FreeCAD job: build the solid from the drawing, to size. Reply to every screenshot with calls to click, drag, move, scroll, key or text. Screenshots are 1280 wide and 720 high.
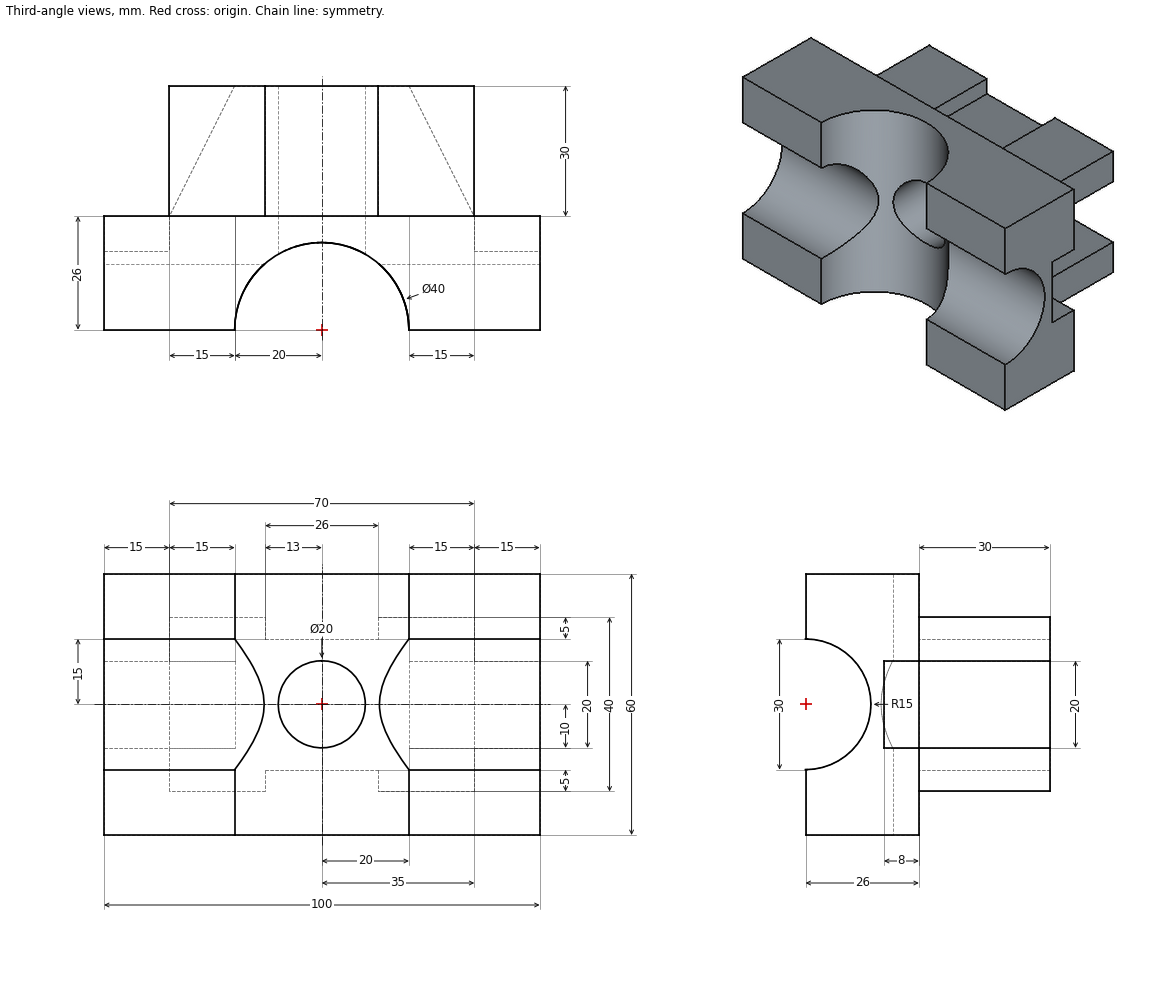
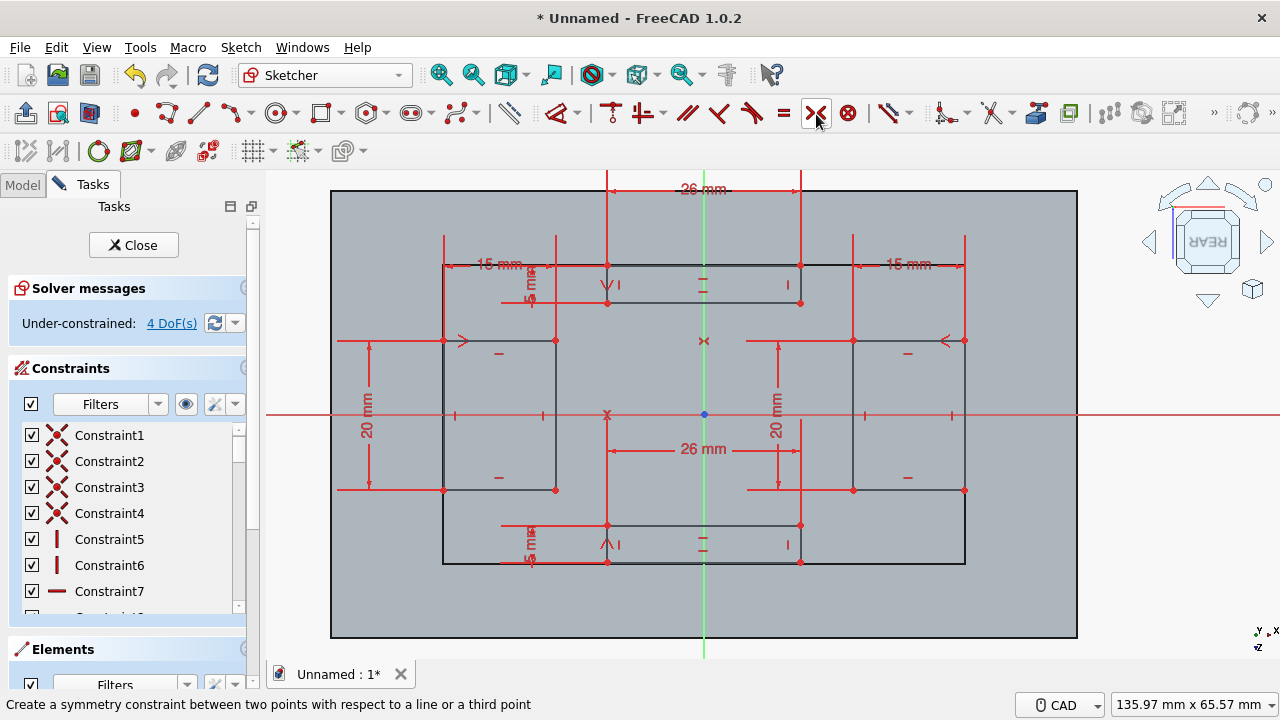
key(d)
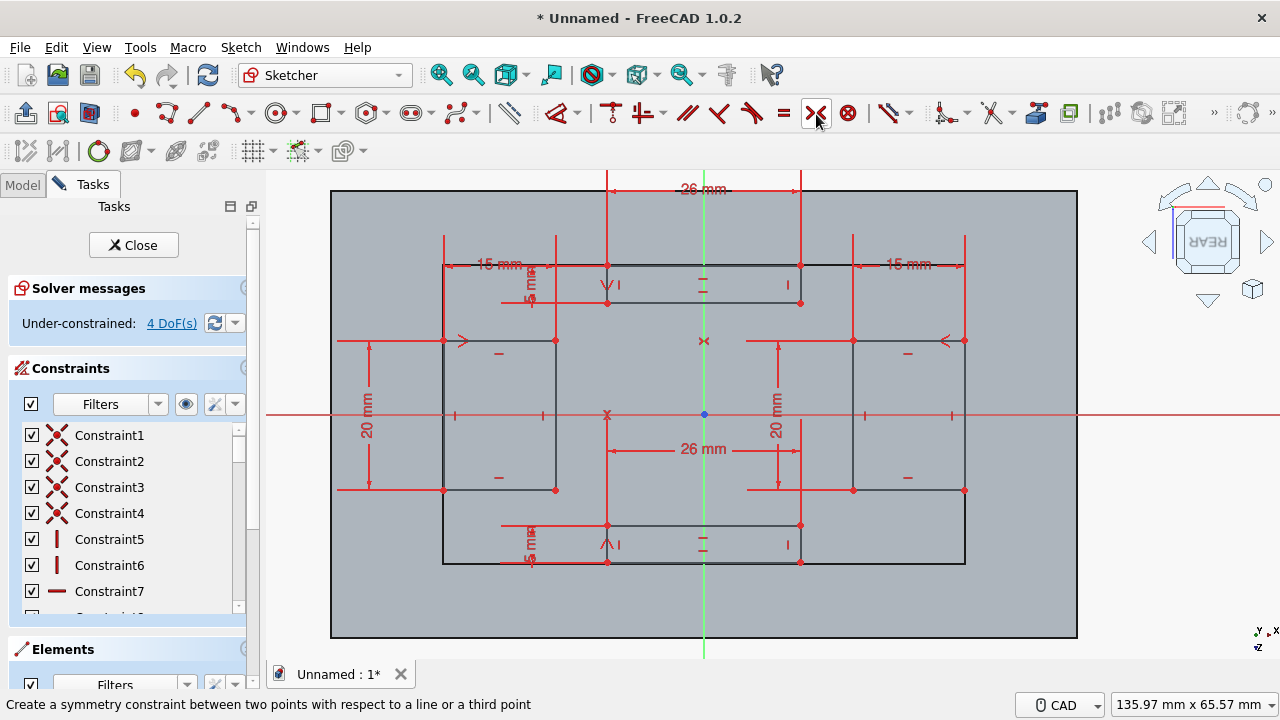
click(853, 341)
click(831, 307)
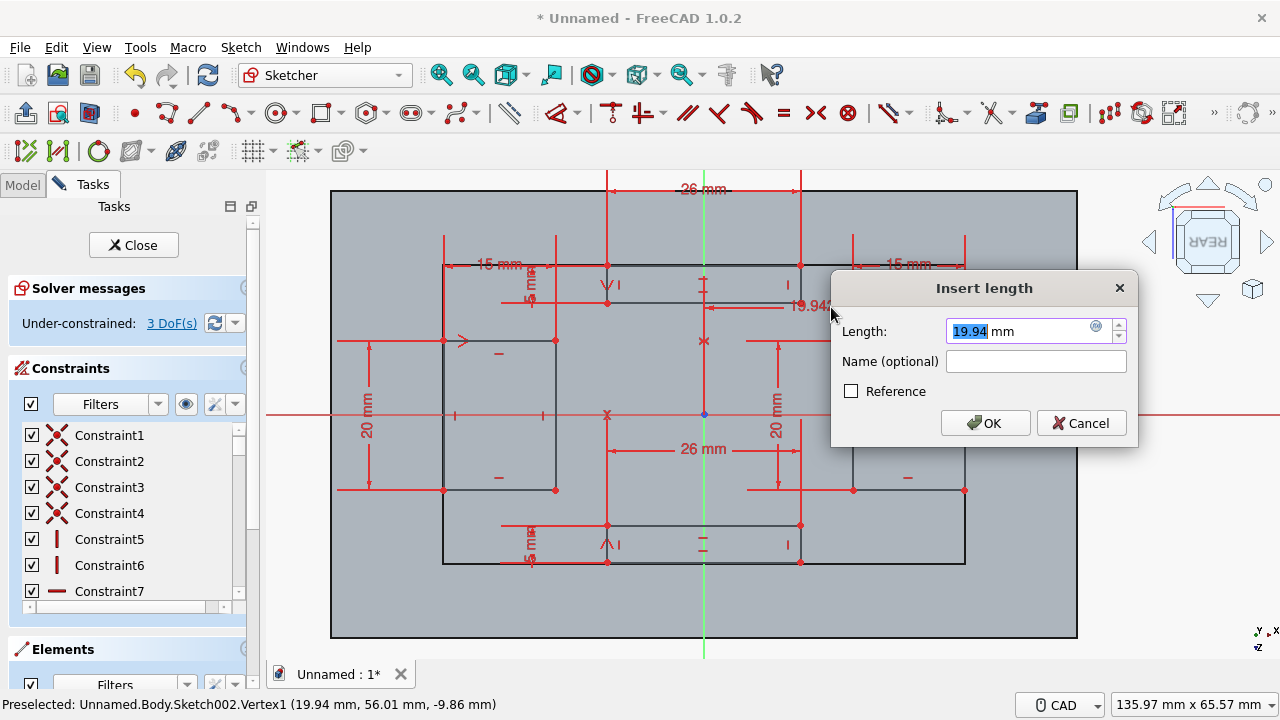
text(20)
key(Return)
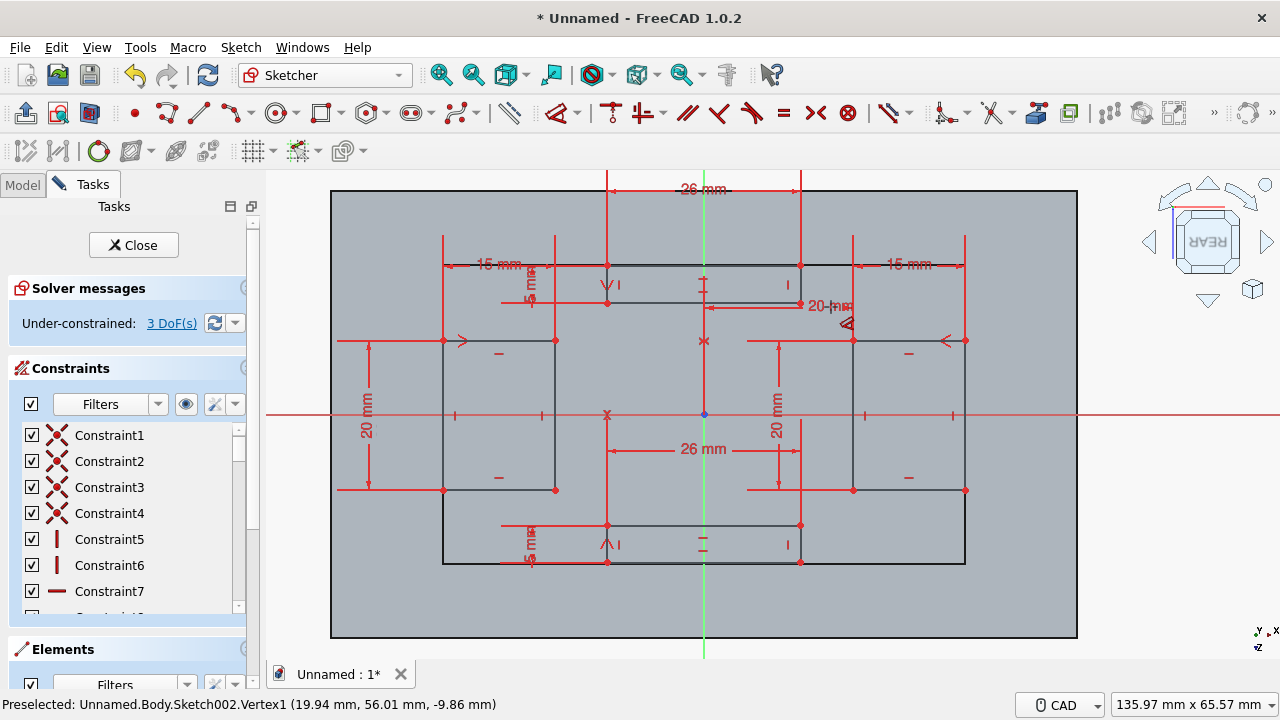
click(853, 341)
click(887, 378)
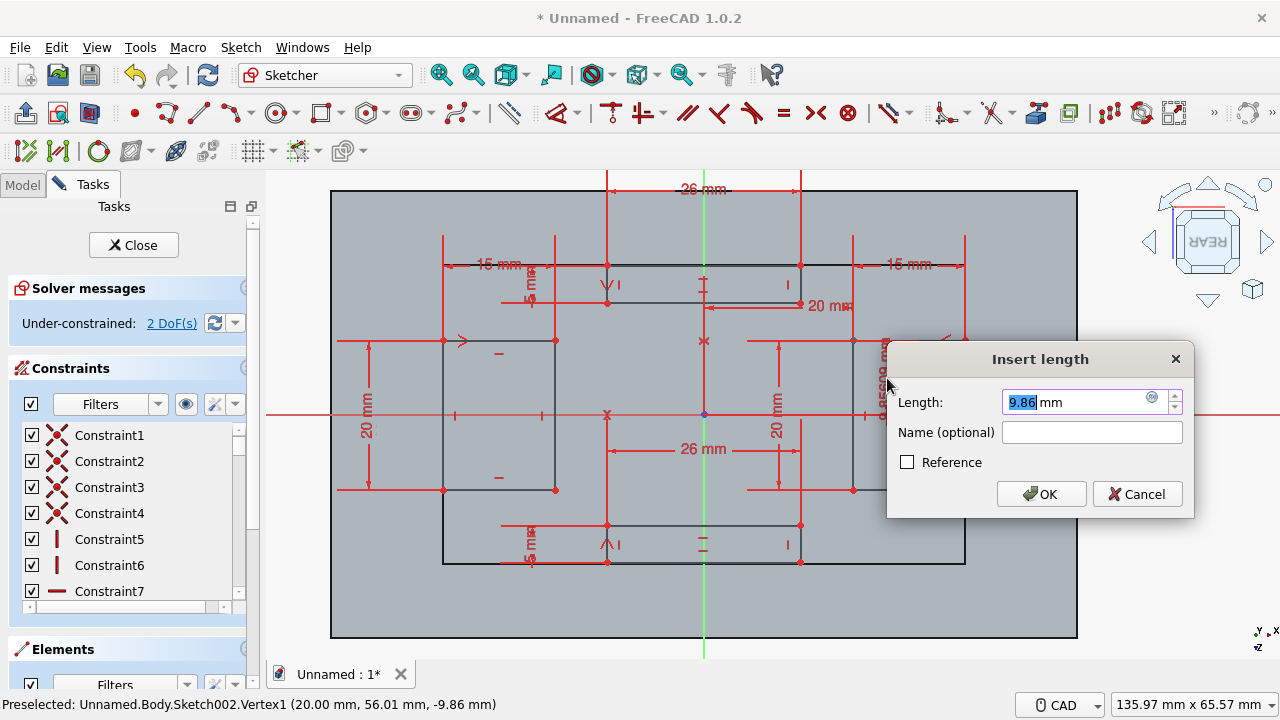
text(10)
key(Return)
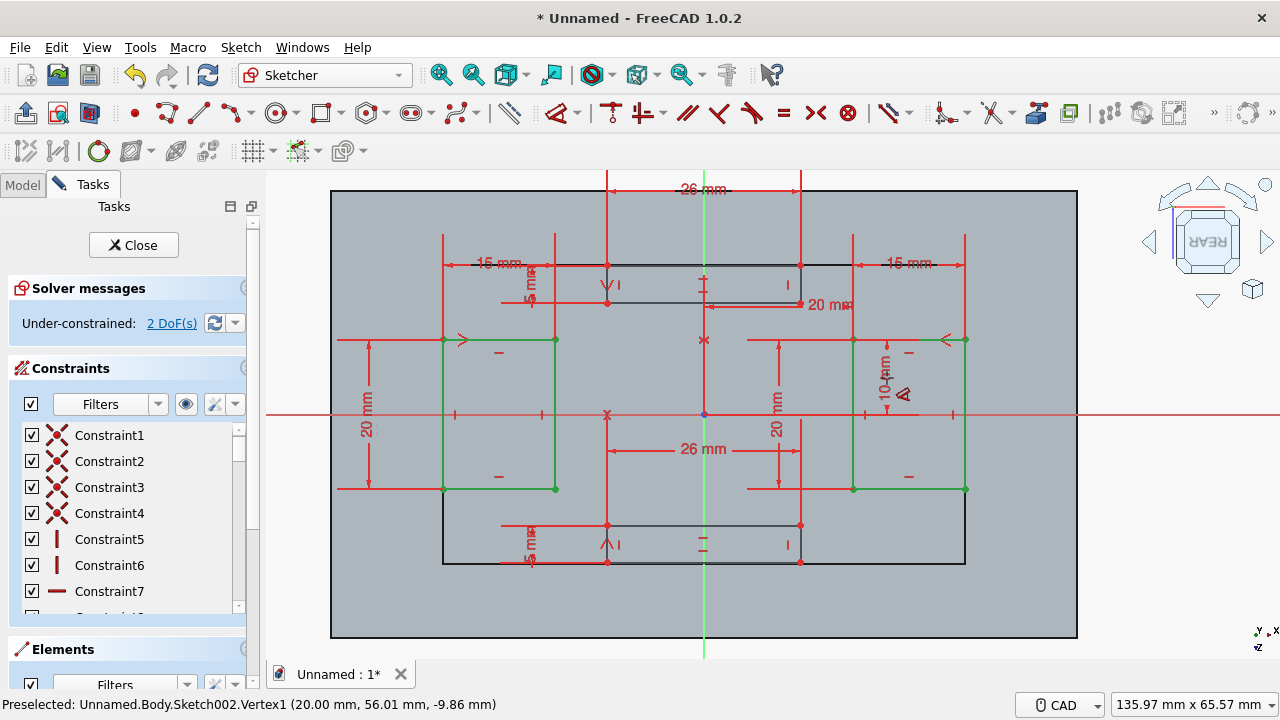
click(607, 526)
click(656, 380)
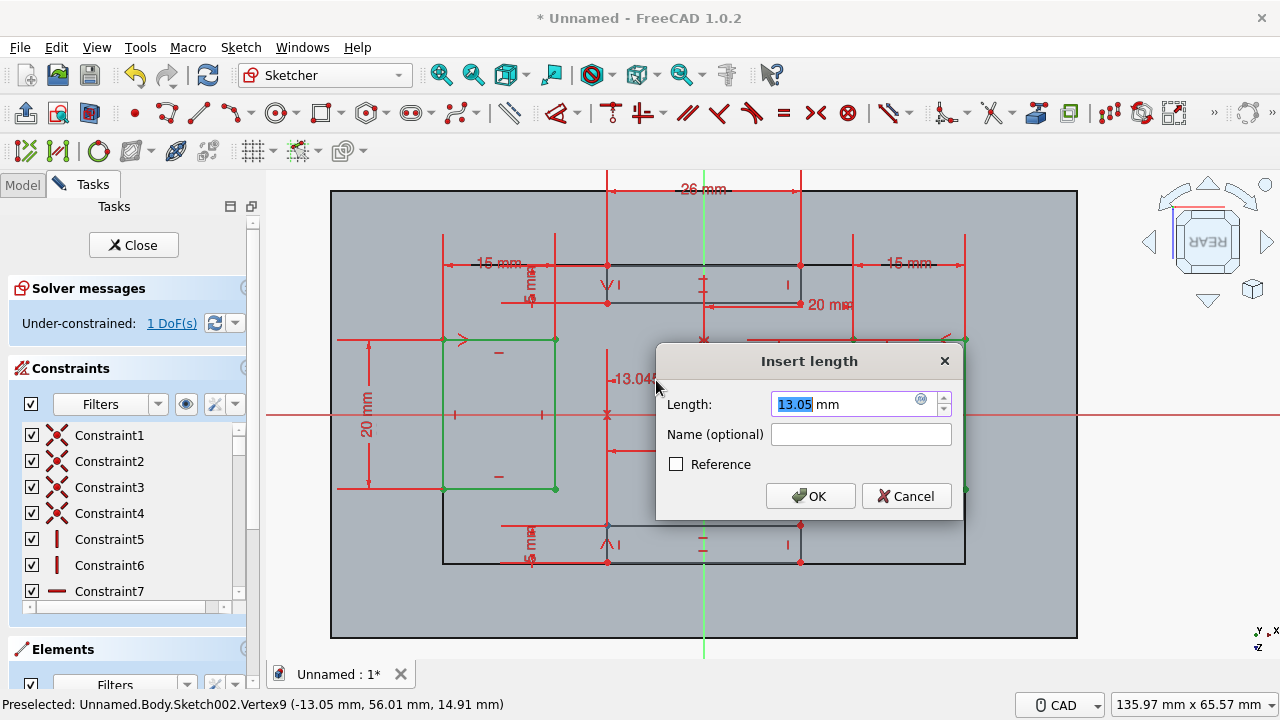
text(13)
key(Return)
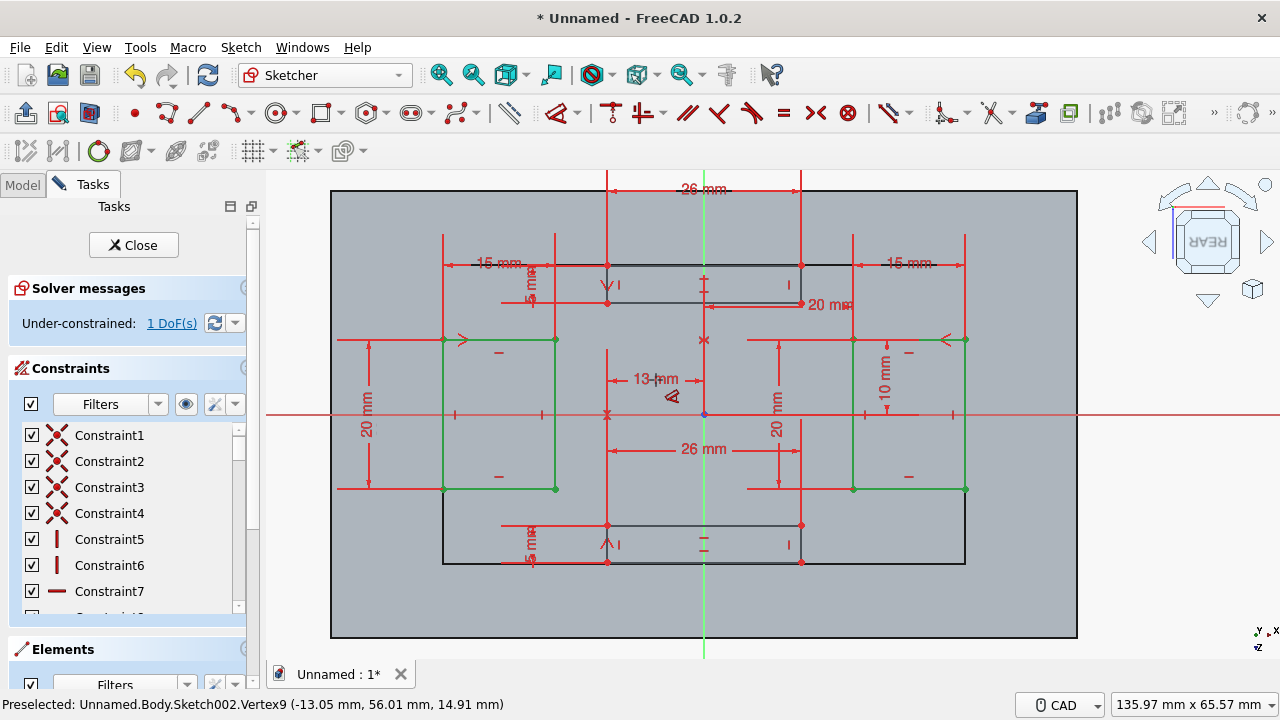
click(607, 526)
click(573, 470)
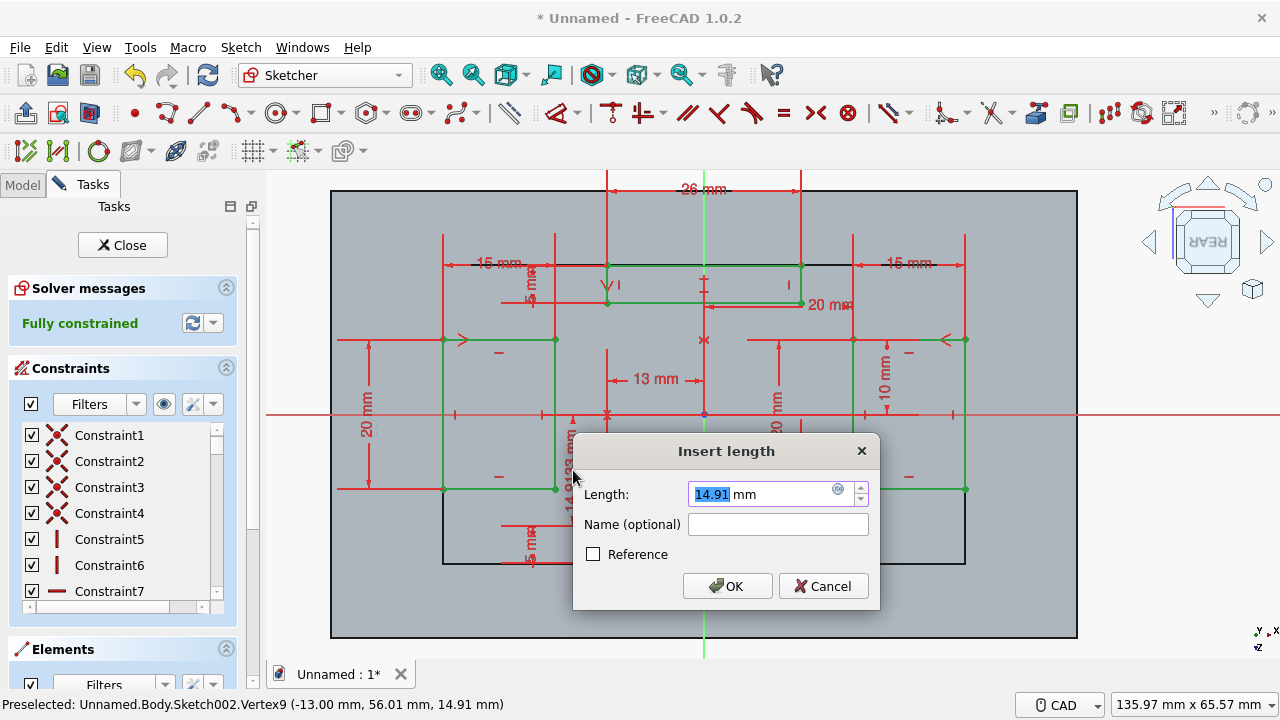
text(15)
key(Return)
key(Escape)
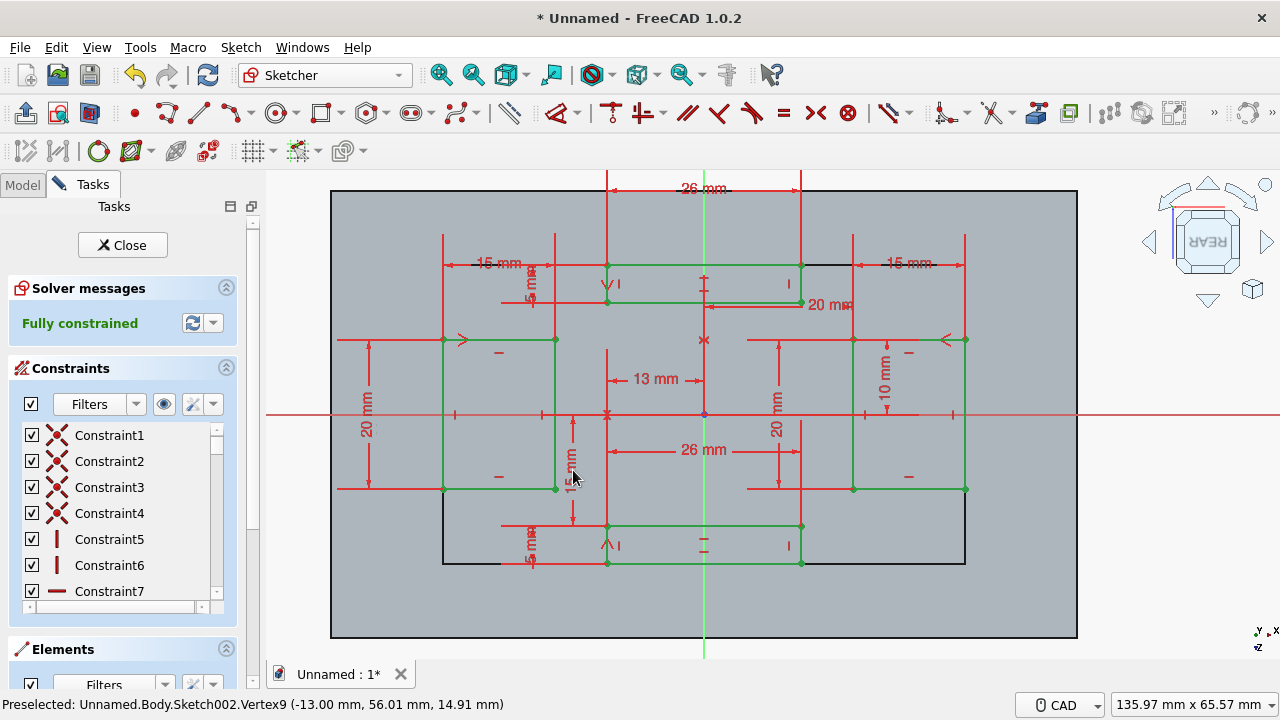
click(123, 245)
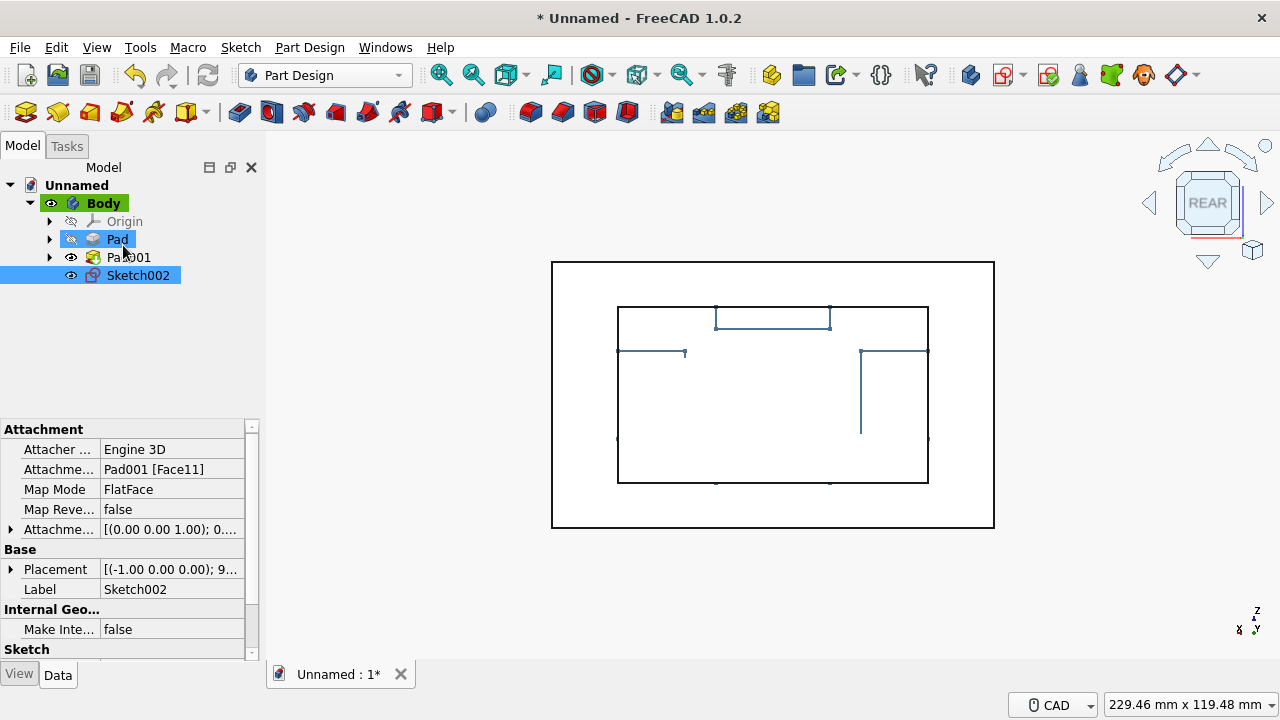
click(240, 112)